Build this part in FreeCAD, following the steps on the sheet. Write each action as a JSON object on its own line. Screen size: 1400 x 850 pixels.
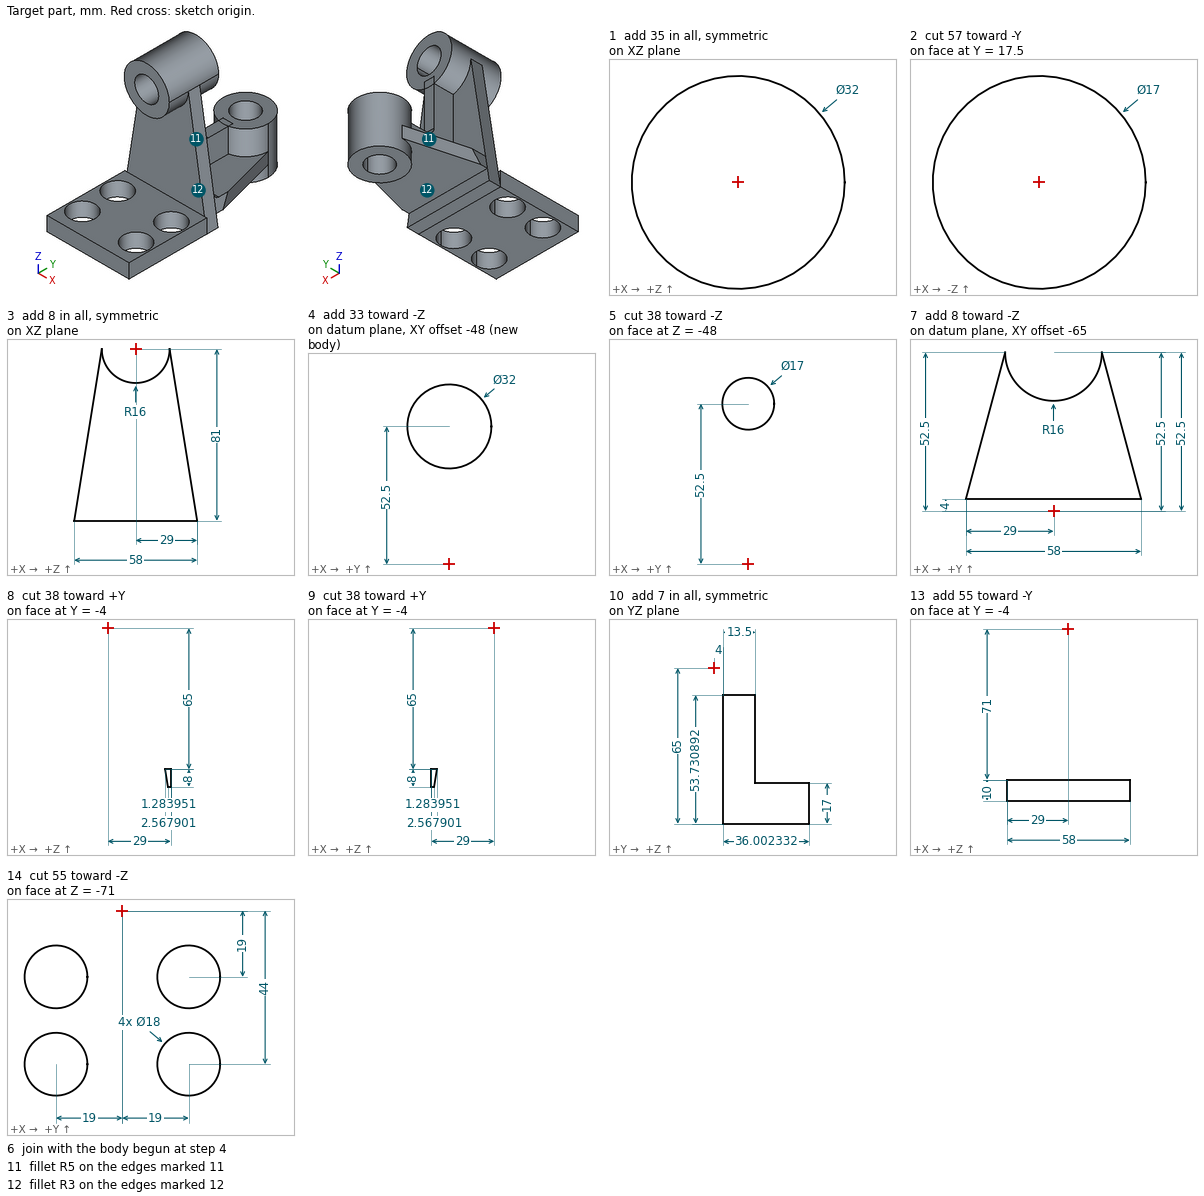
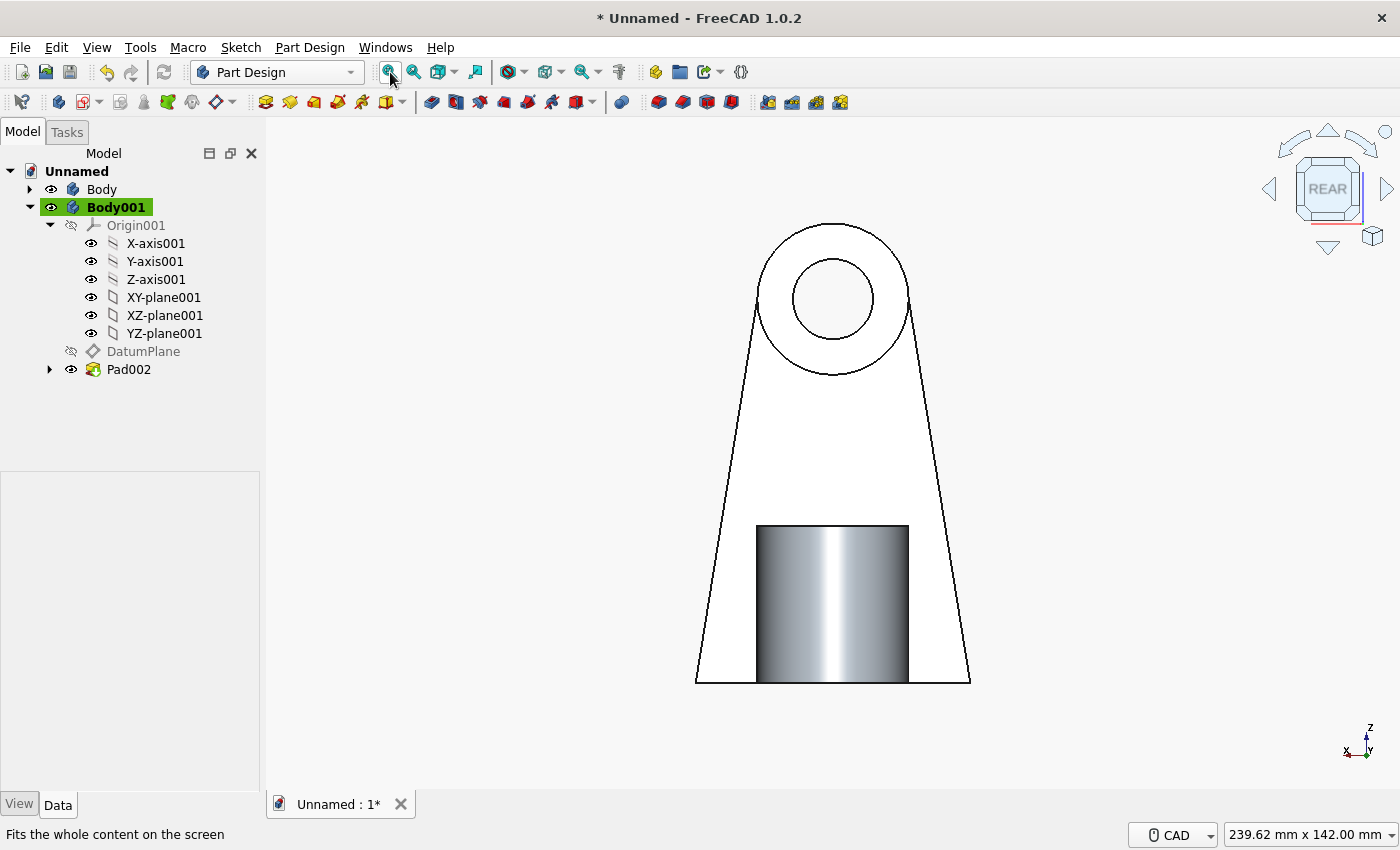
{"action": "key", "text": "0"}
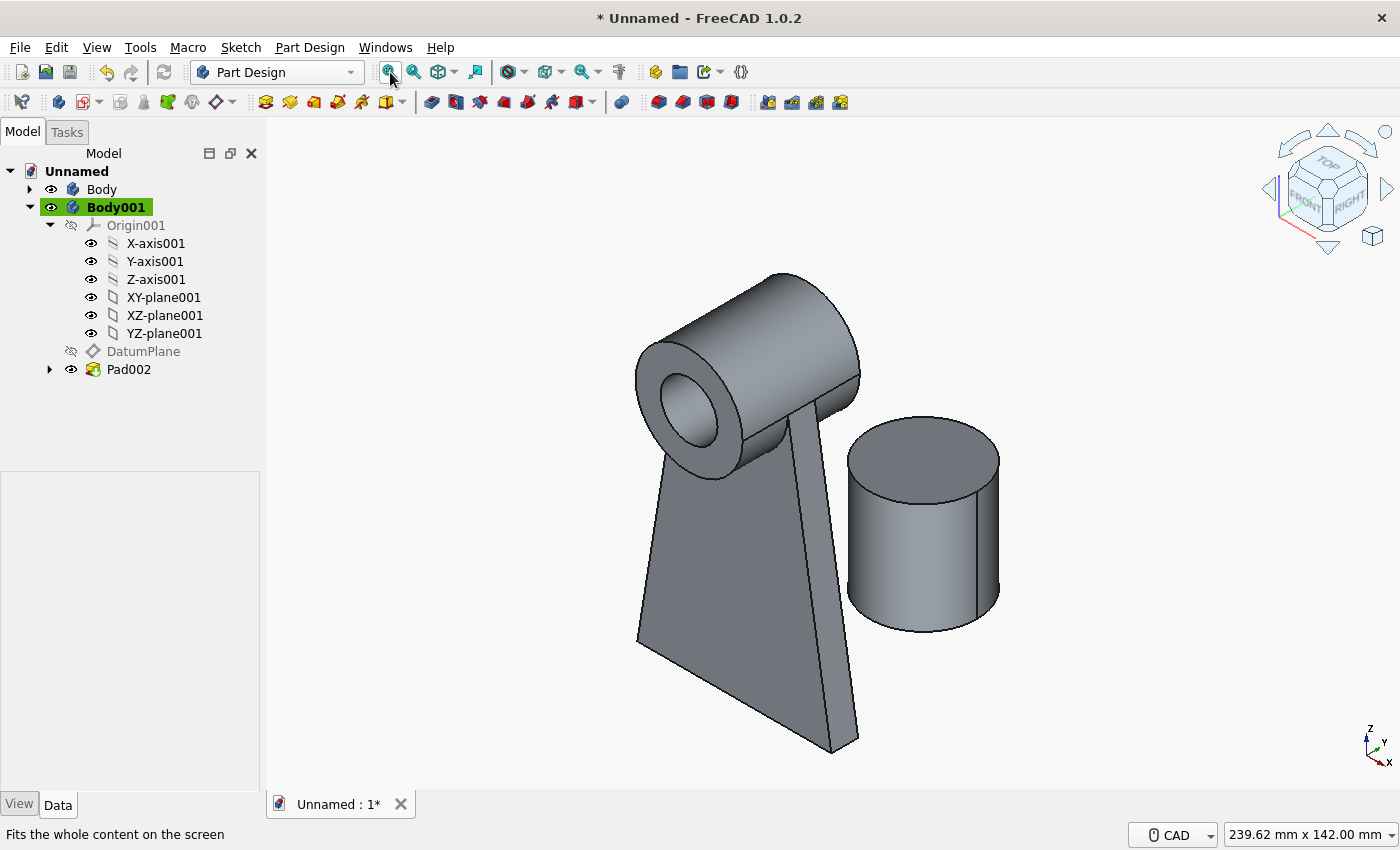
{"action": "key", "text": "v f"}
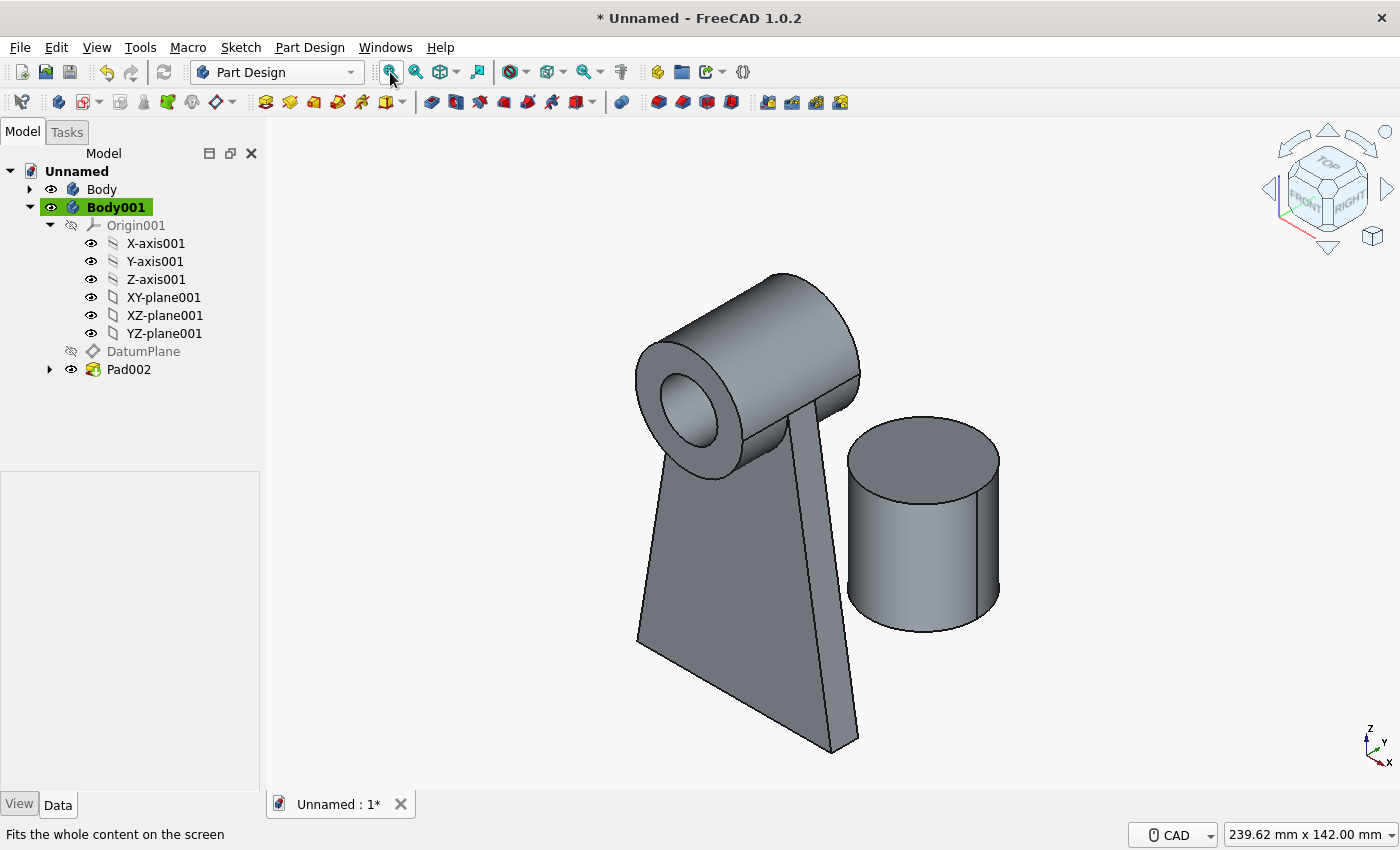
{"action": "left_click", "coordinate": [923, 460]}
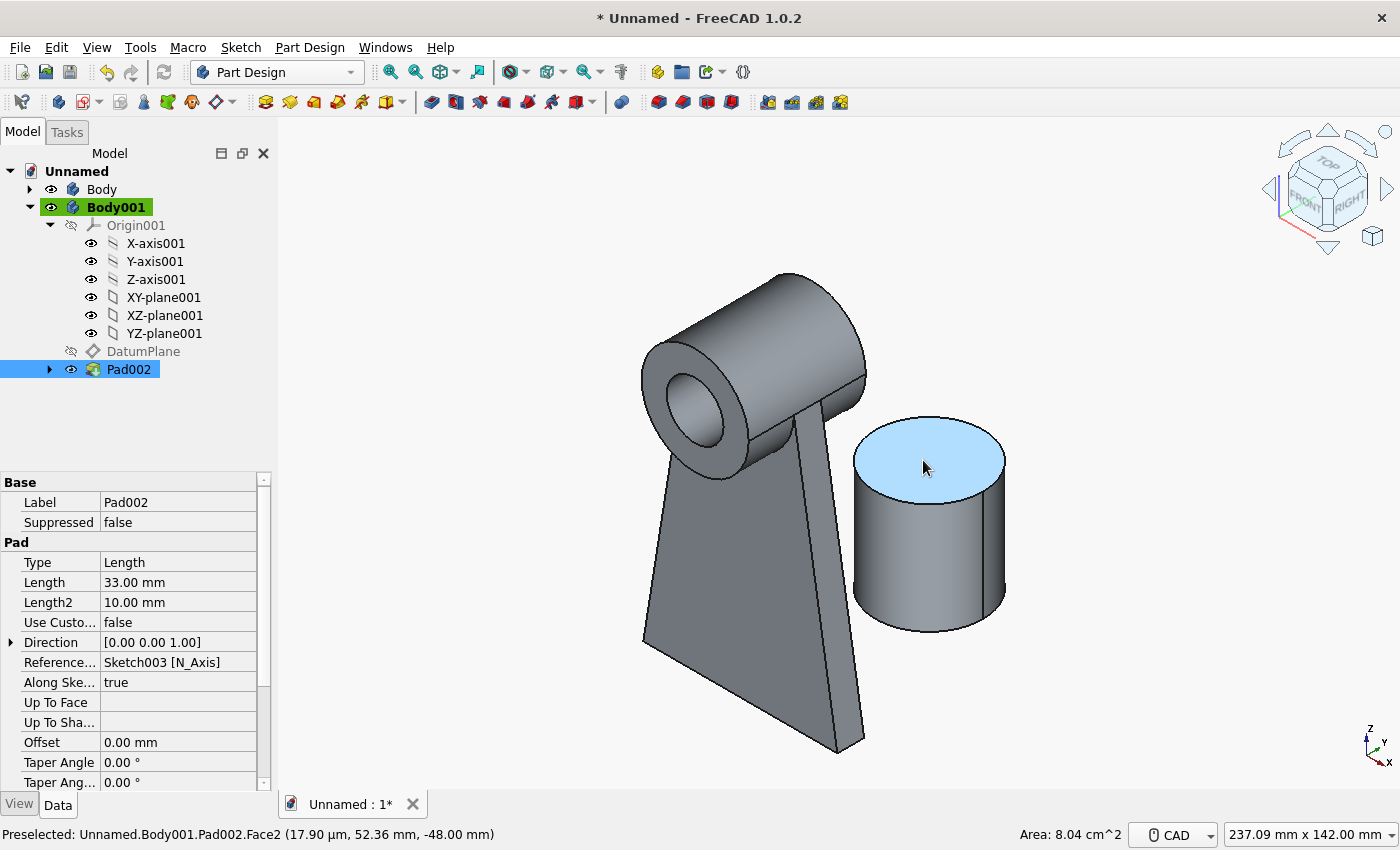
{"action": "left_click", "coordinate": [84, 102]}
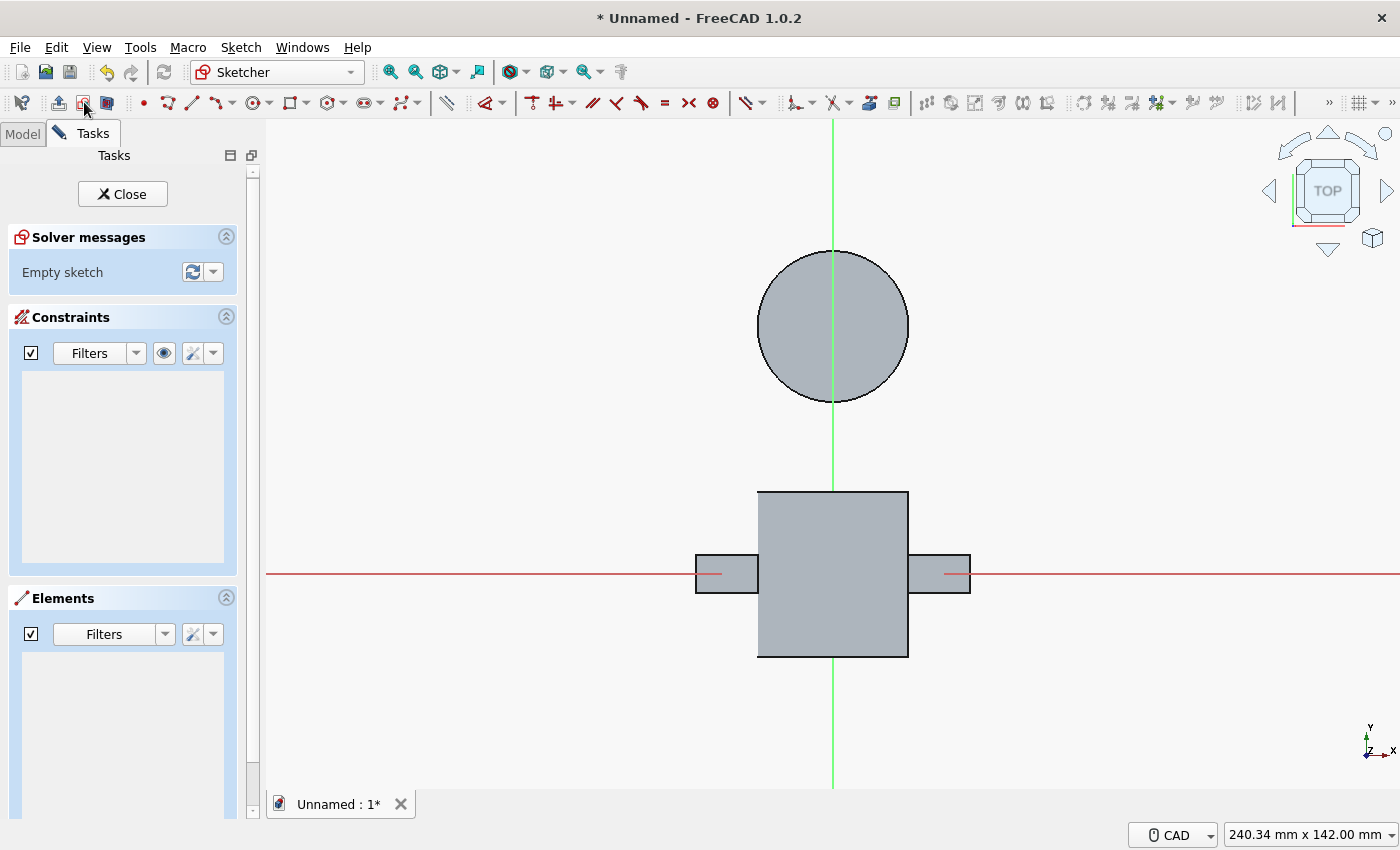
{"action": "scroll", "coordinate": [850, 294], "scroll_direction": "up", "scroll_amount": 8}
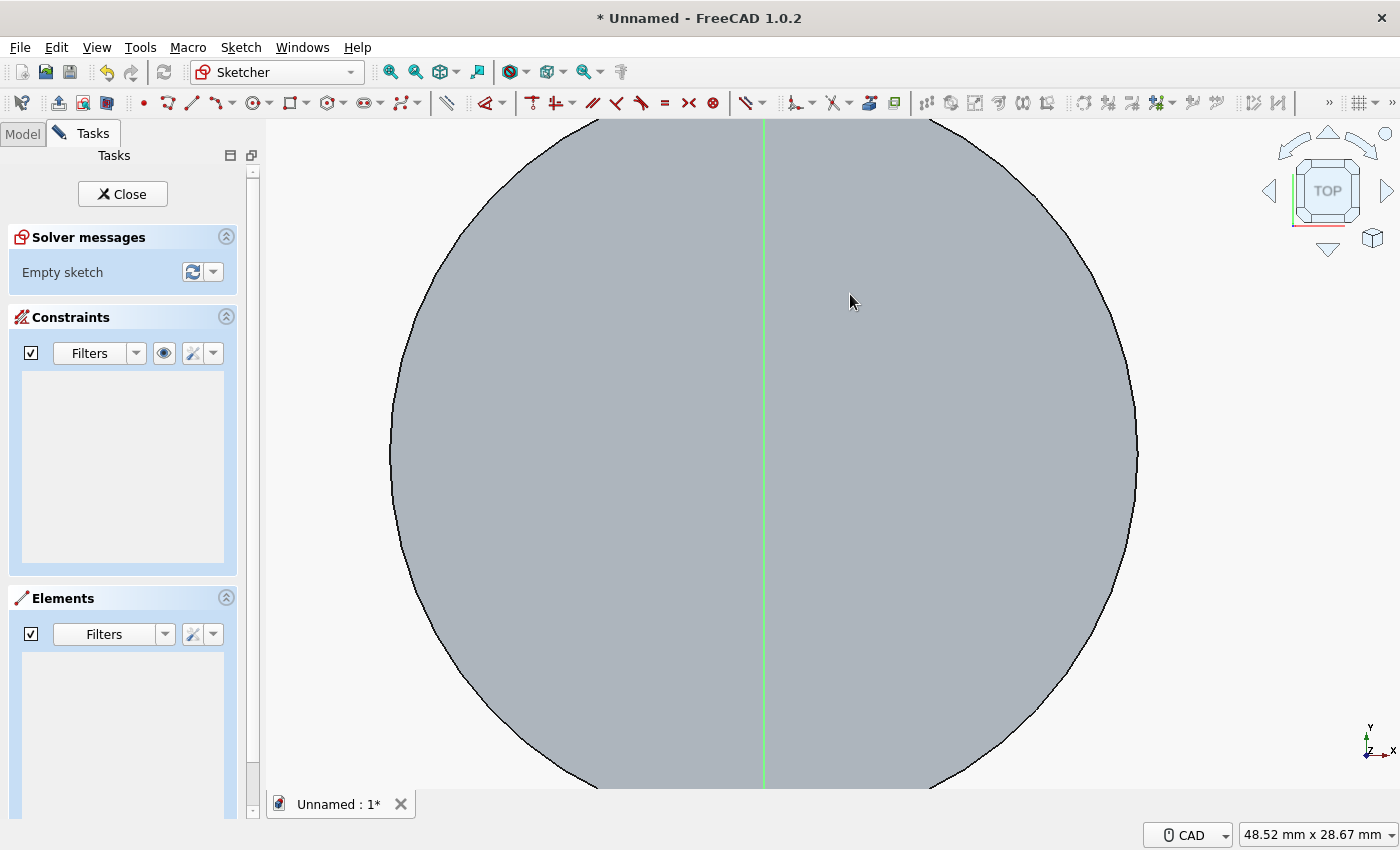
{"action": "key", "text": "g c"}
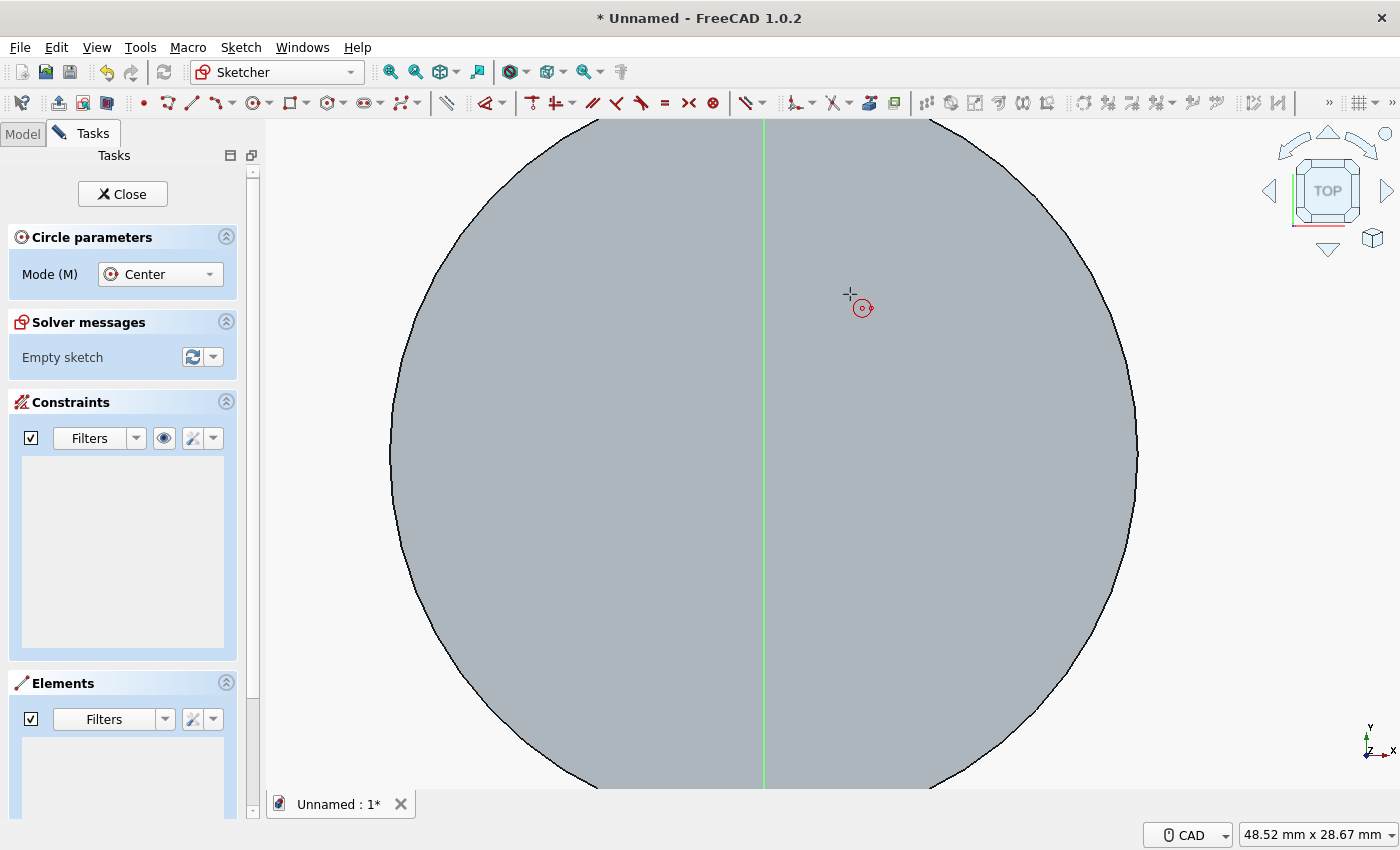
{"action": "left_click", "coordinate": [764, 454]}
{"action": "left_click", "coordinate": [904, 314]}
{"action": "key", "text": "Escape"}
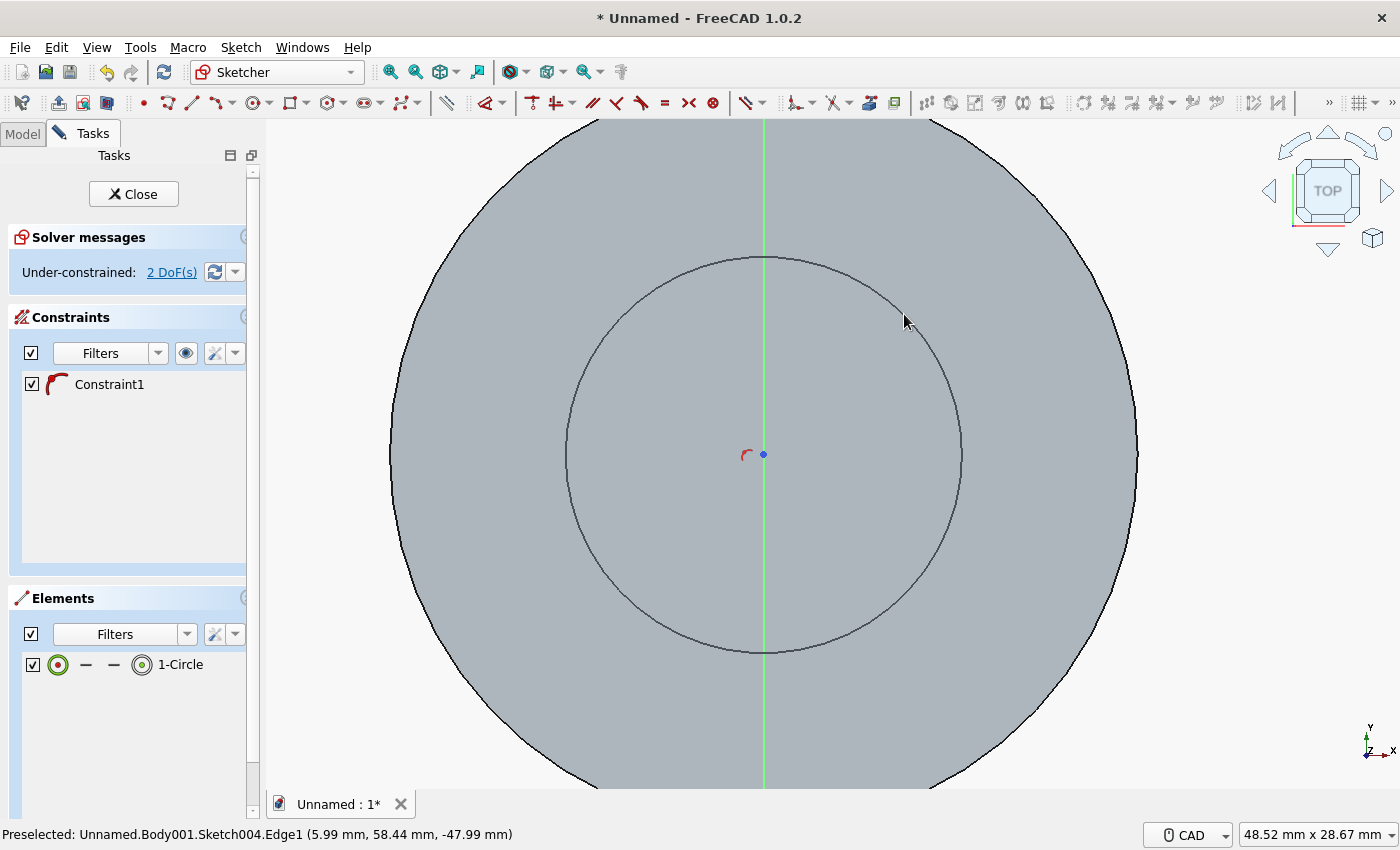
{"action": "left_click", "coordinate": [486, 104]}